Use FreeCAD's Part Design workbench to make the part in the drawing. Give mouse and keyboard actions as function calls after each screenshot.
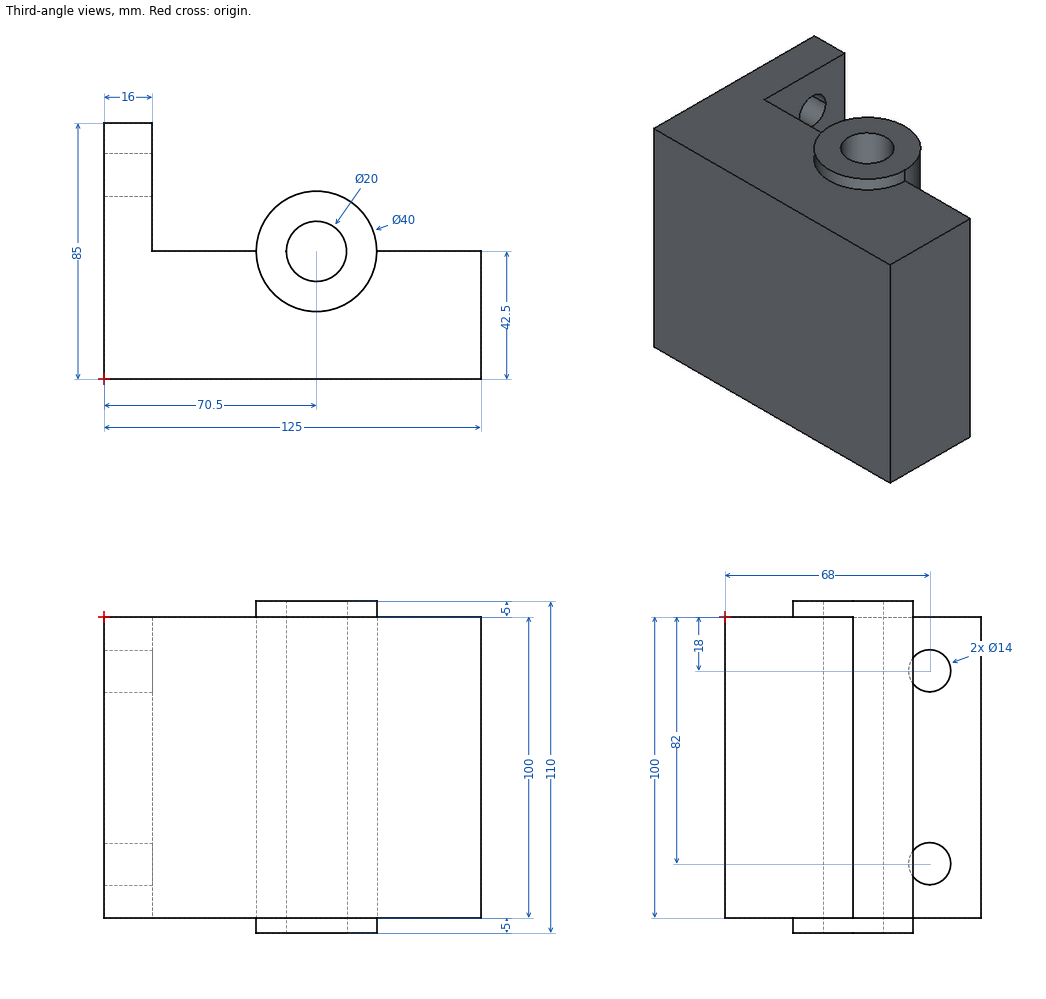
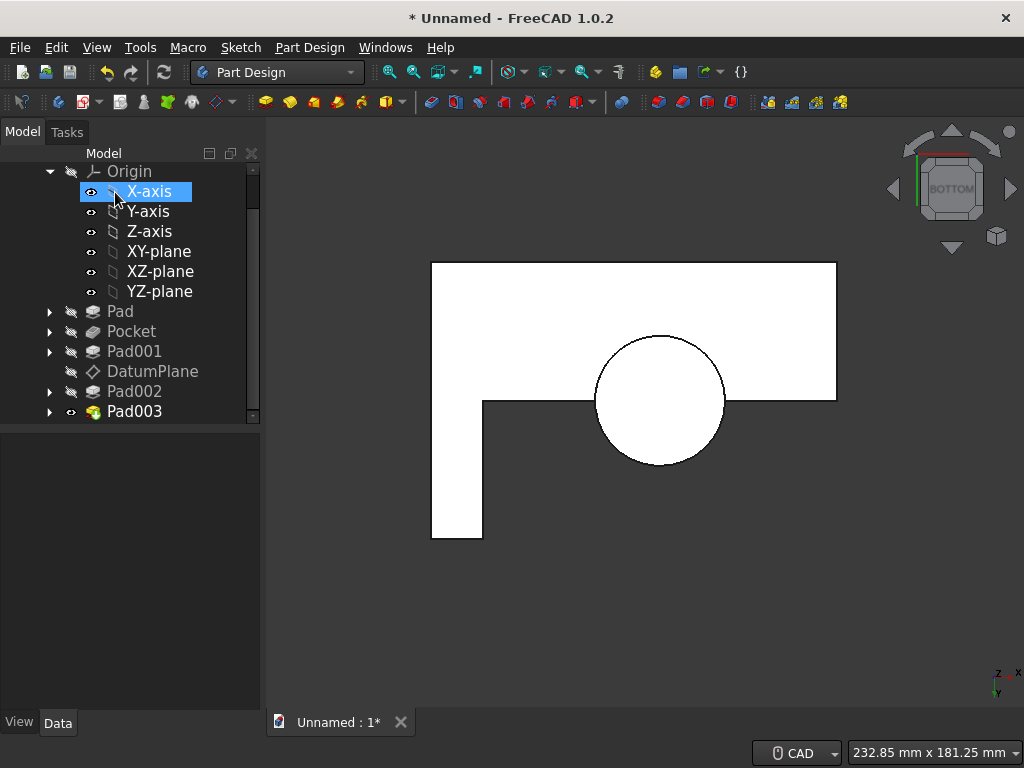
click(660, 400)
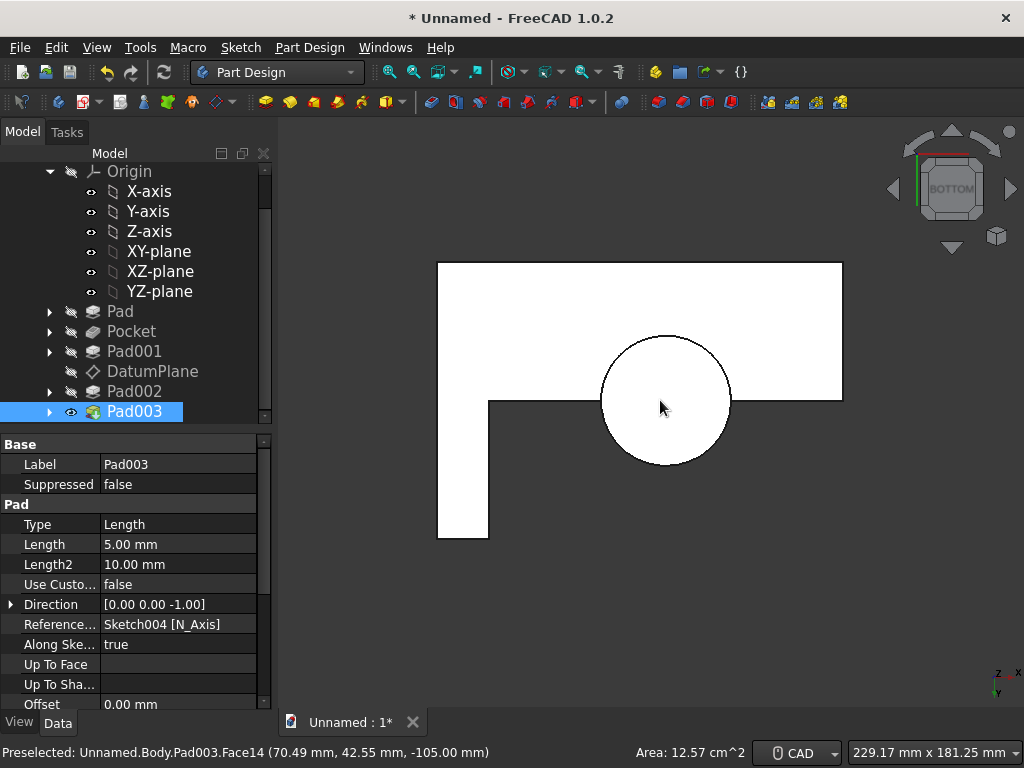
click(84, 102)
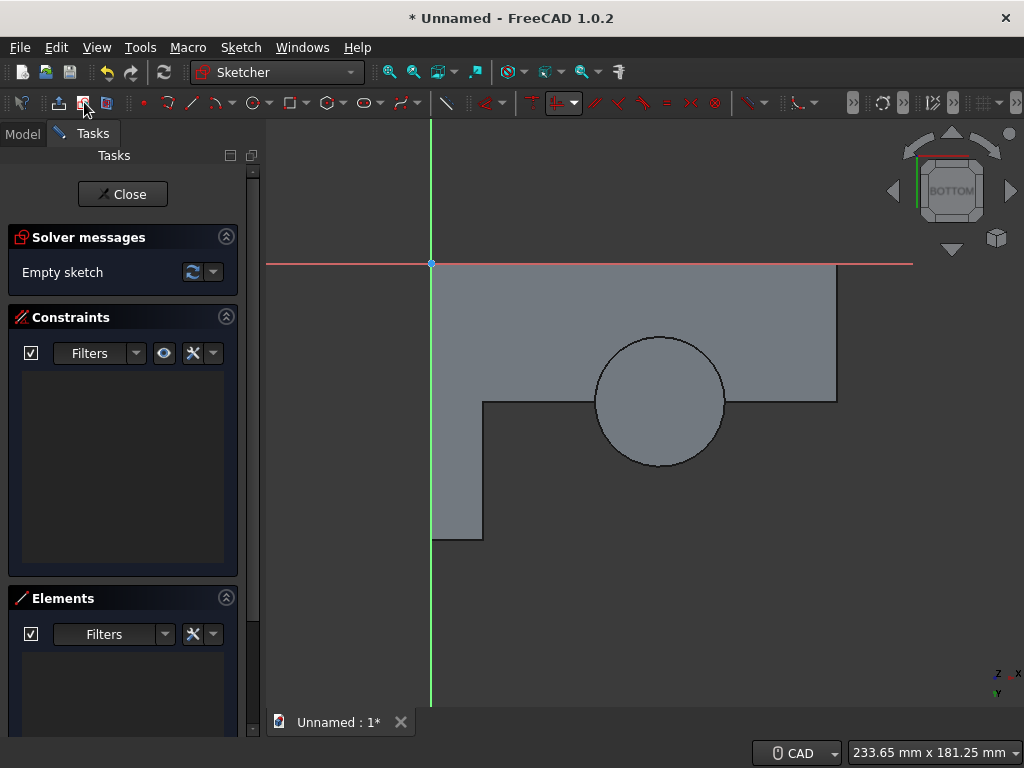
scroll(677, 400, up, 9)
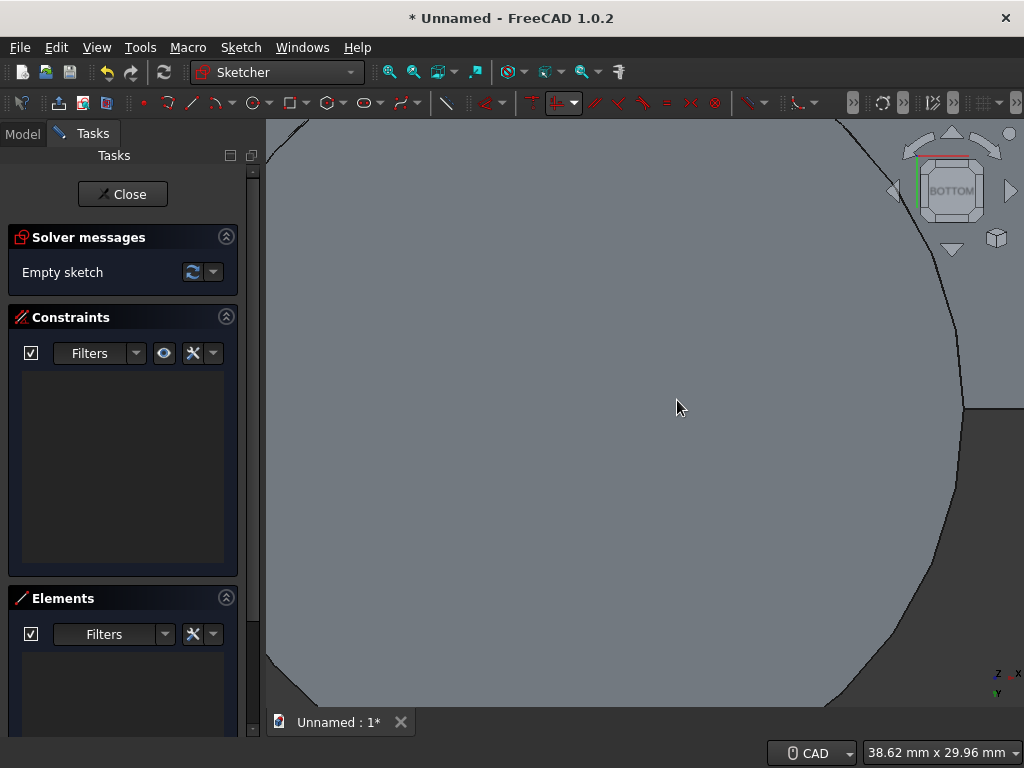
key(g)
key(c)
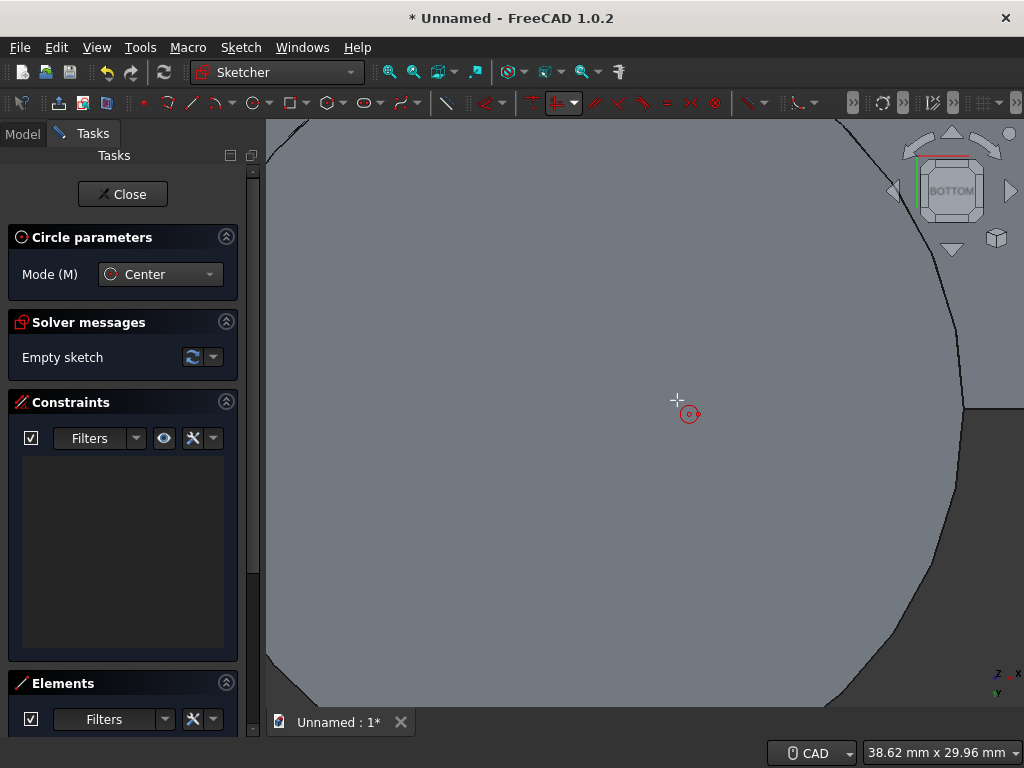
click(571, 409)
move(710, 270)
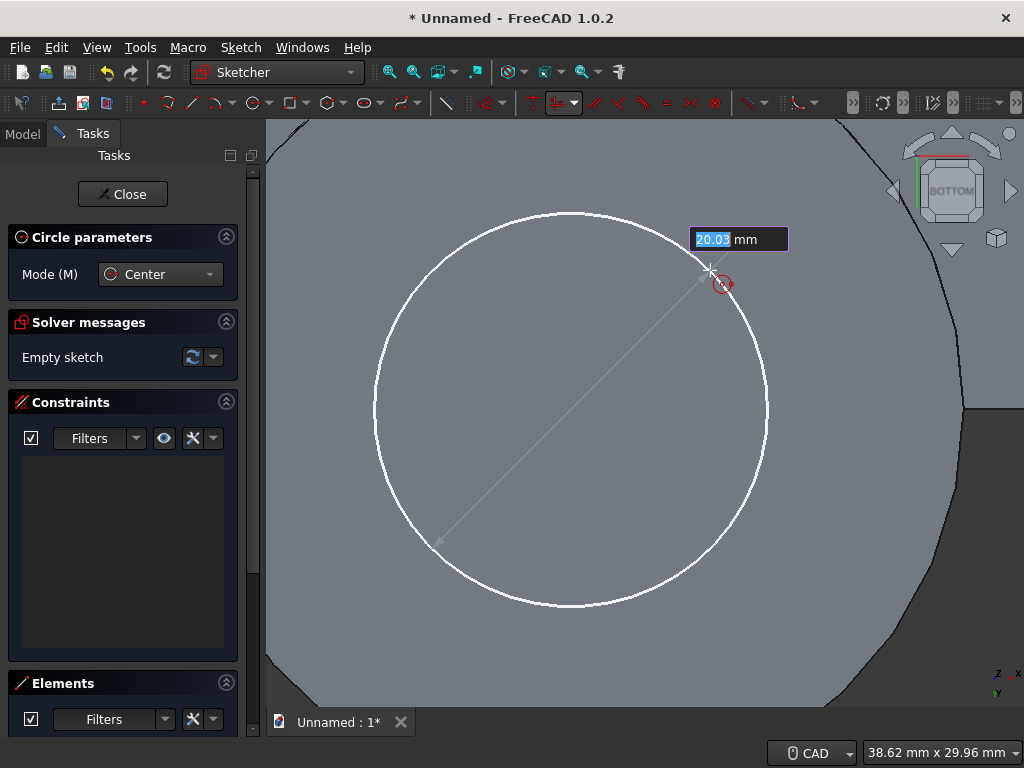
text(20)
key(Return)
key(Escape)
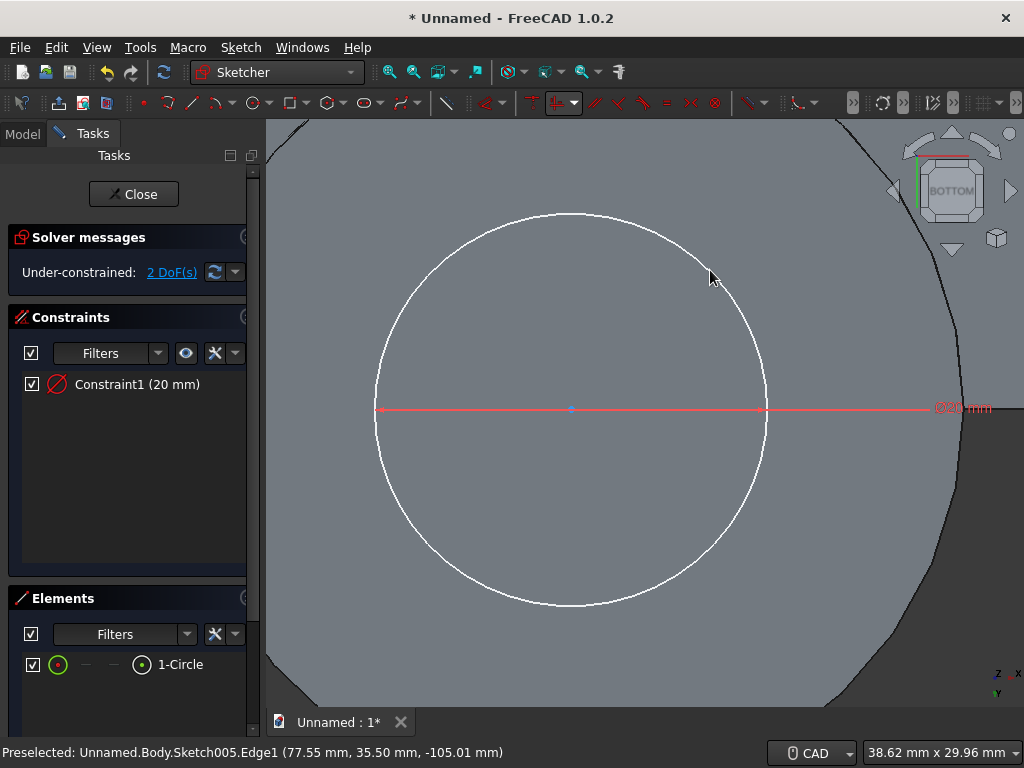
click(486, 104)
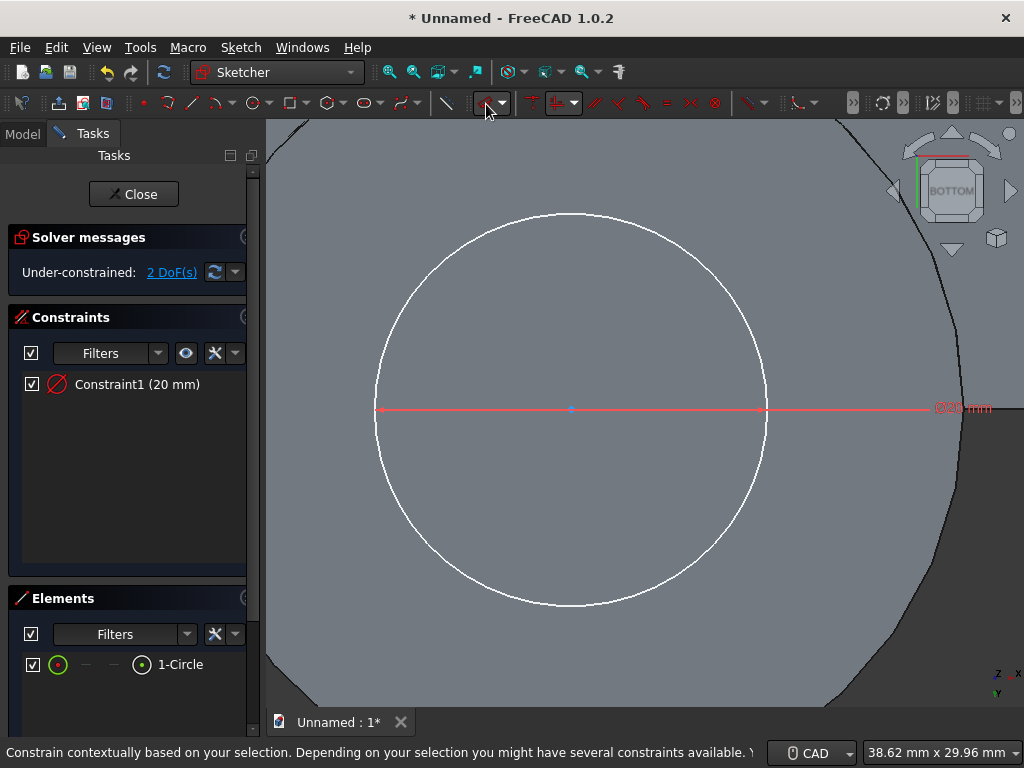
click(571, 410)
click(433, 444)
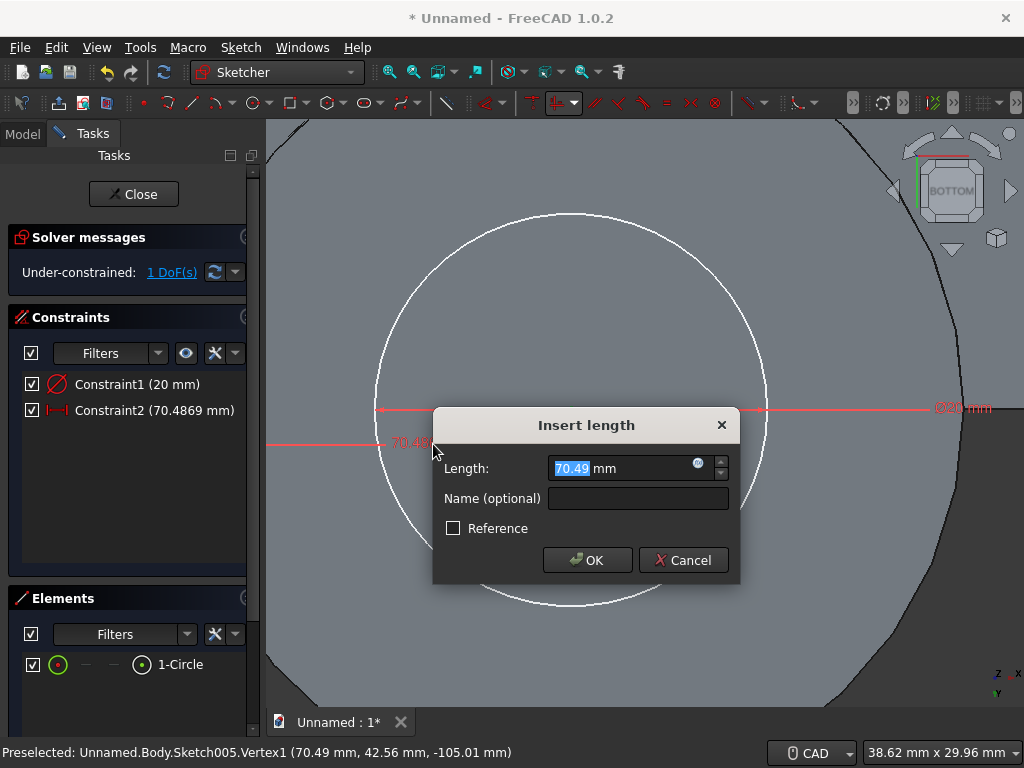
text(70.5)
key(Return)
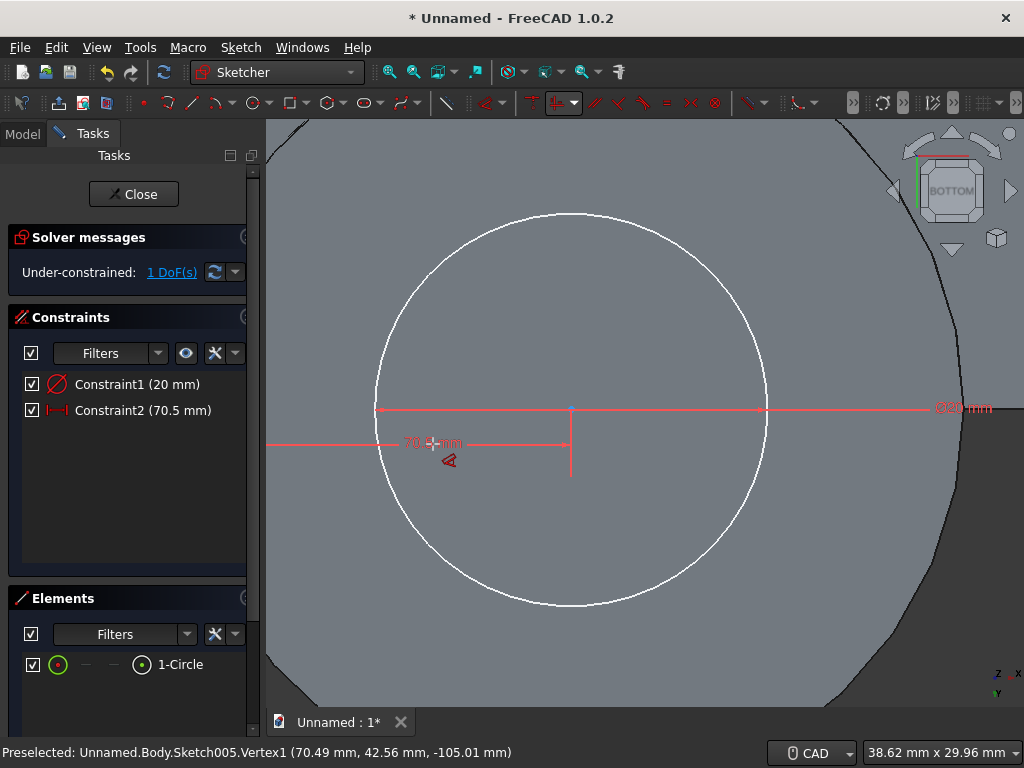
click(571, 410)
click(605, 279)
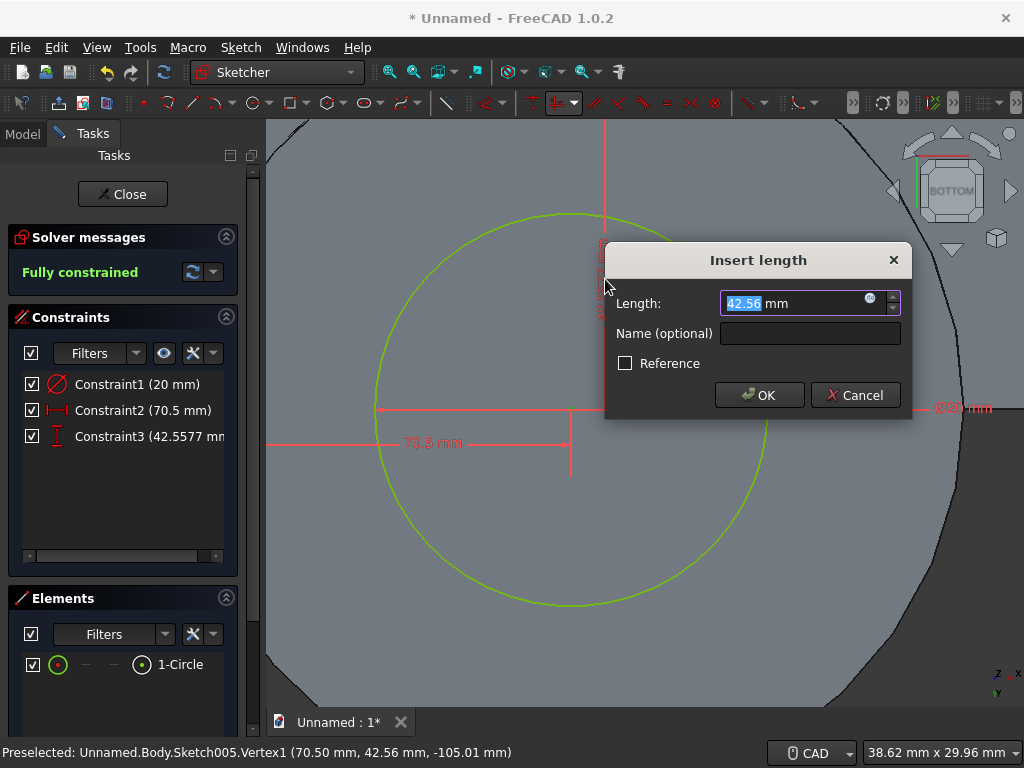
text(42.5)
key(Return)
key(Escape)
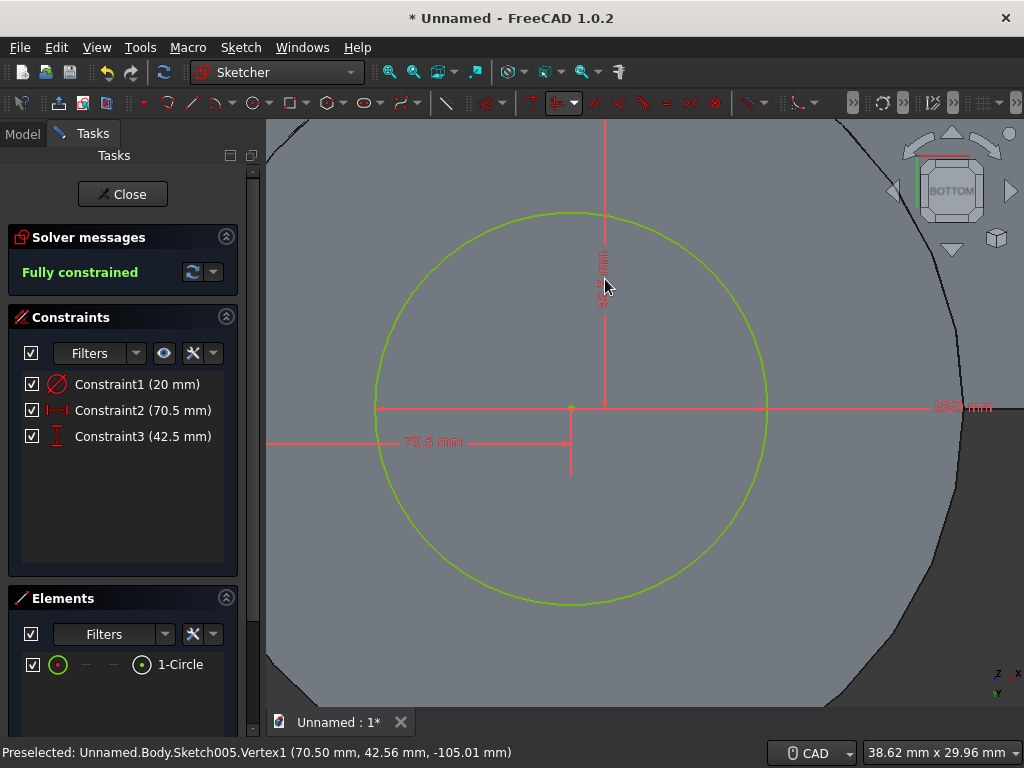
click(123, 194)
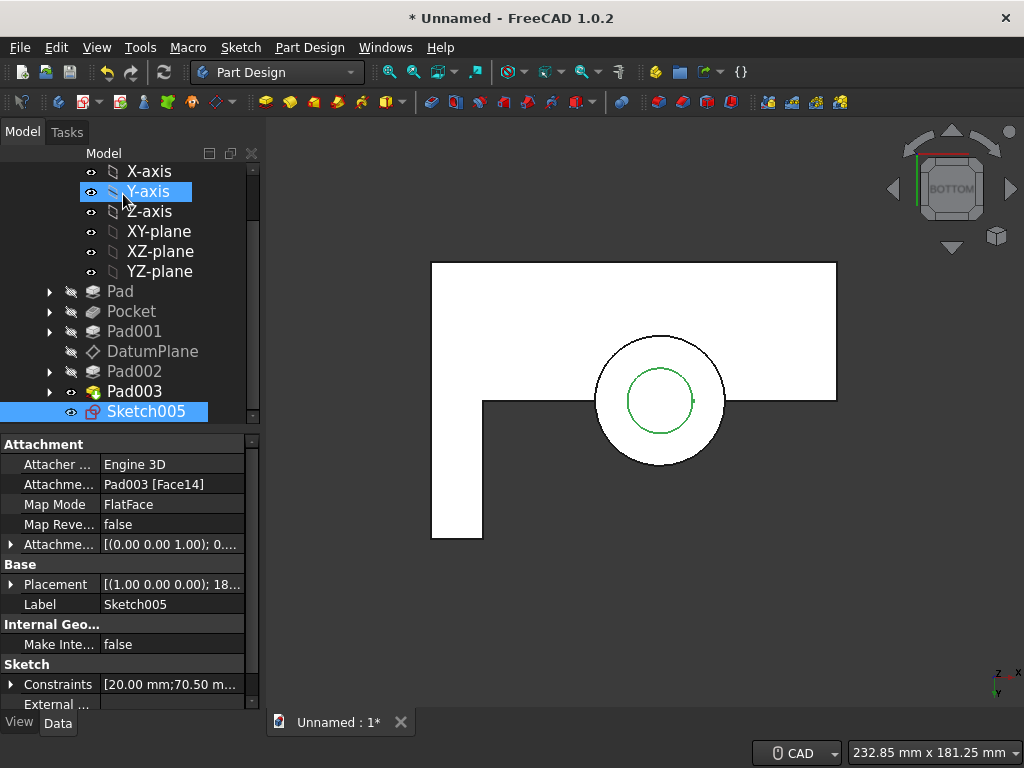
click(432, 102)